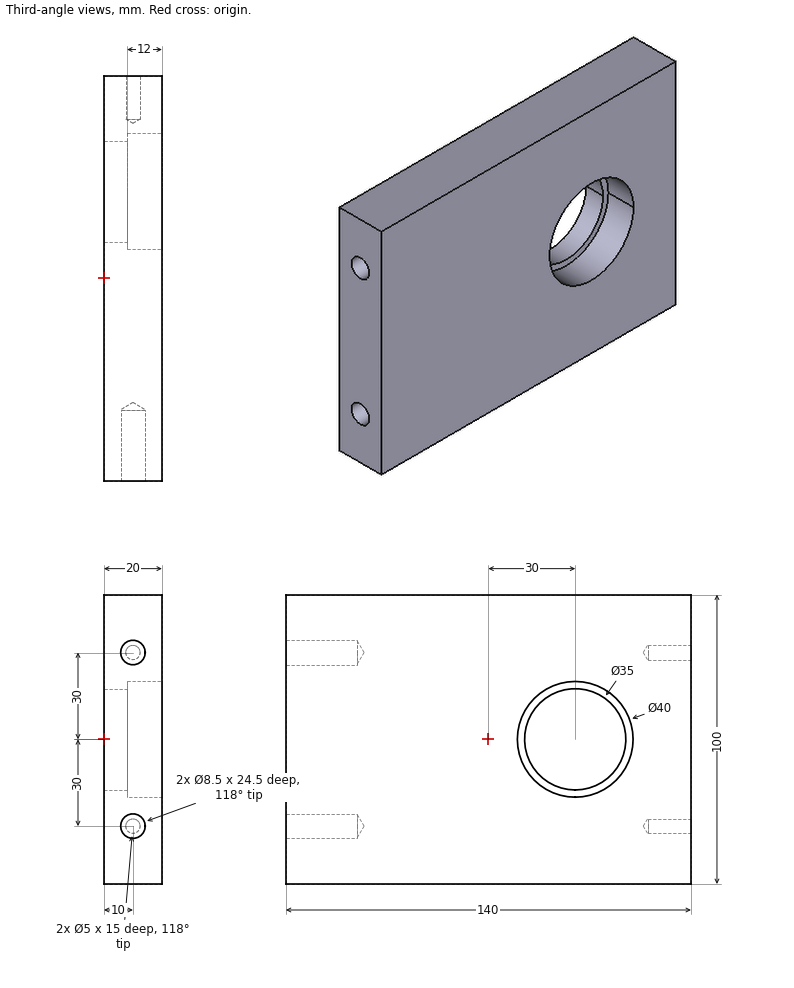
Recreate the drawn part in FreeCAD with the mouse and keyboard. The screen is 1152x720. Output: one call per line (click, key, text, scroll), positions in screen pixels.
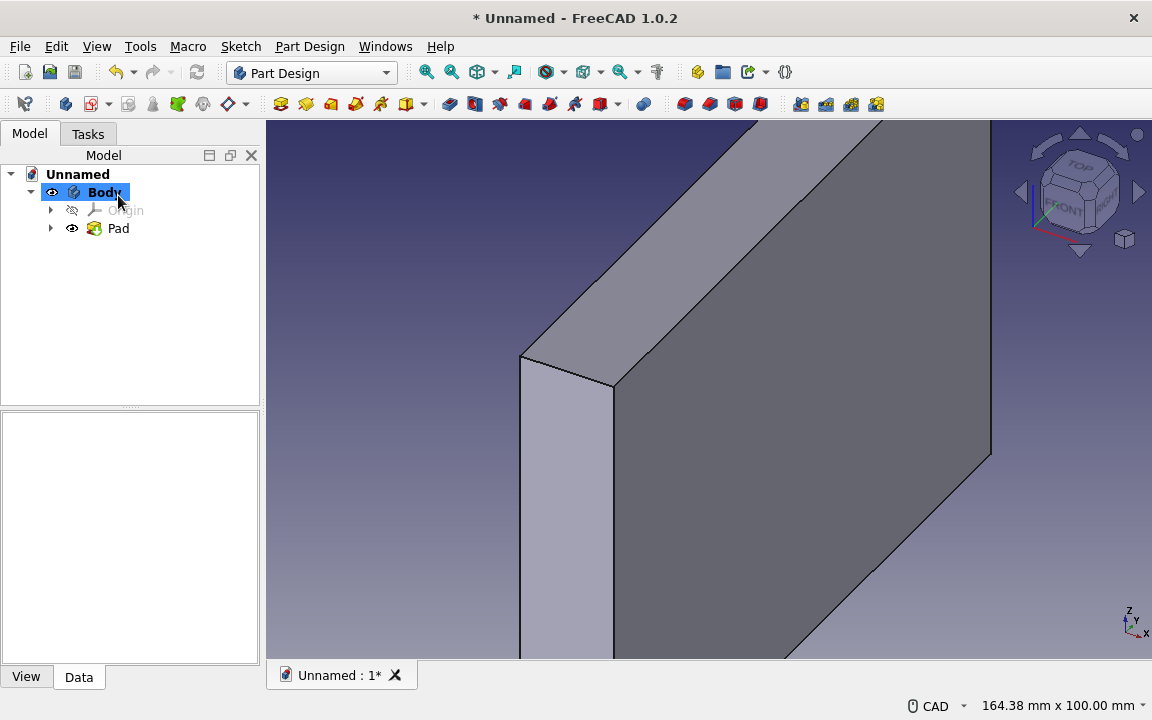
click(427, 72)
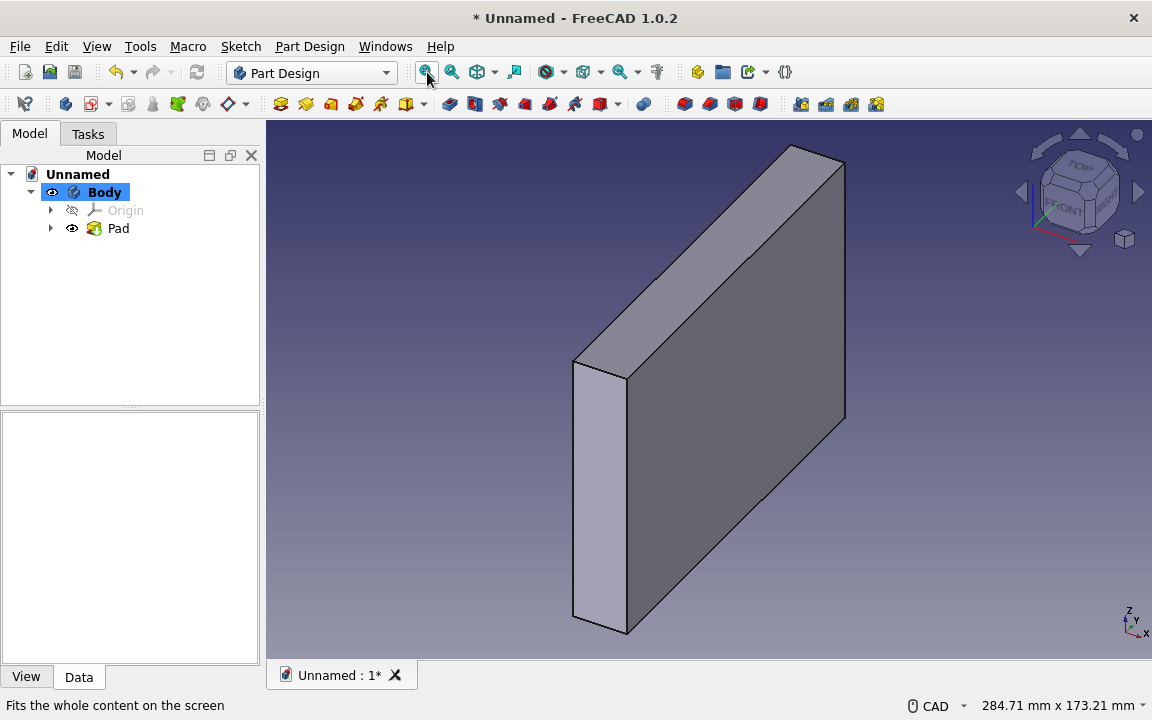
click(600, 497)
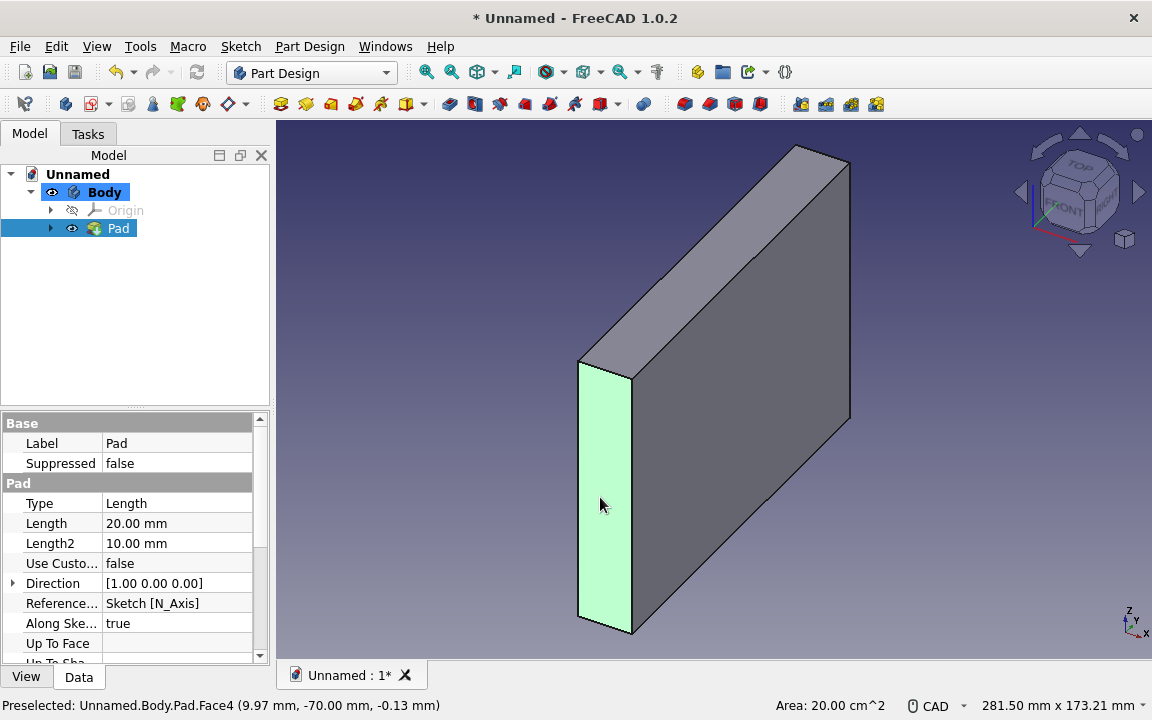
click(90, 104)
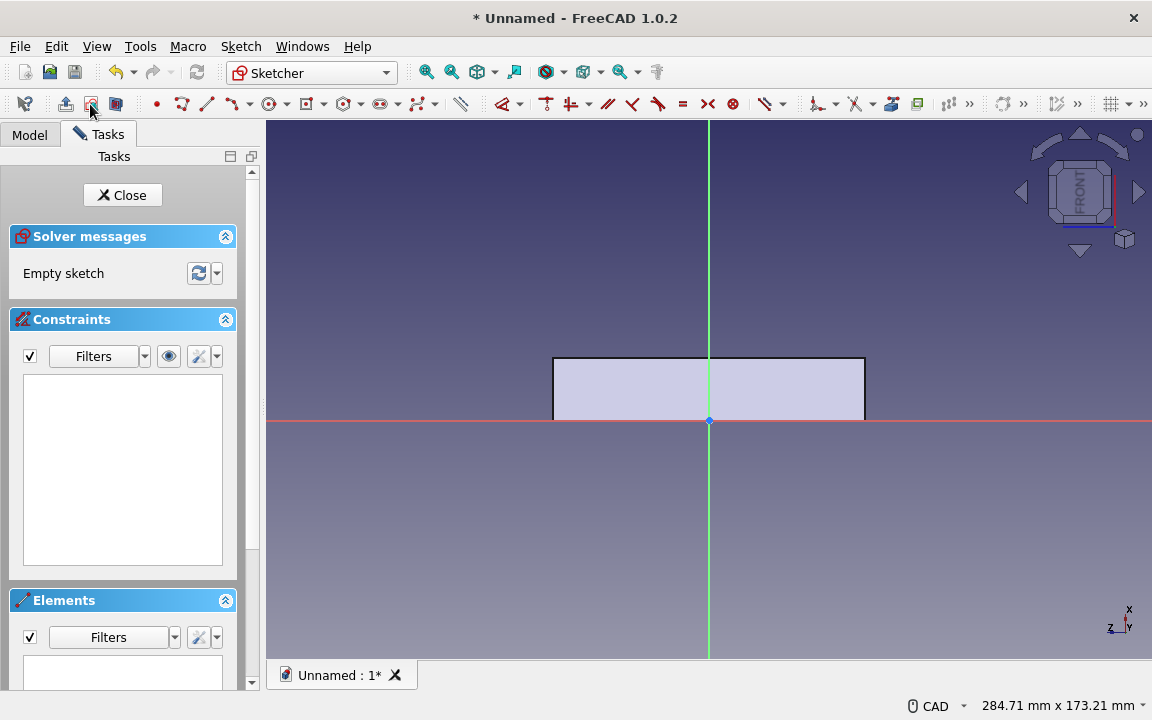
scroll(765, 406, up, 4)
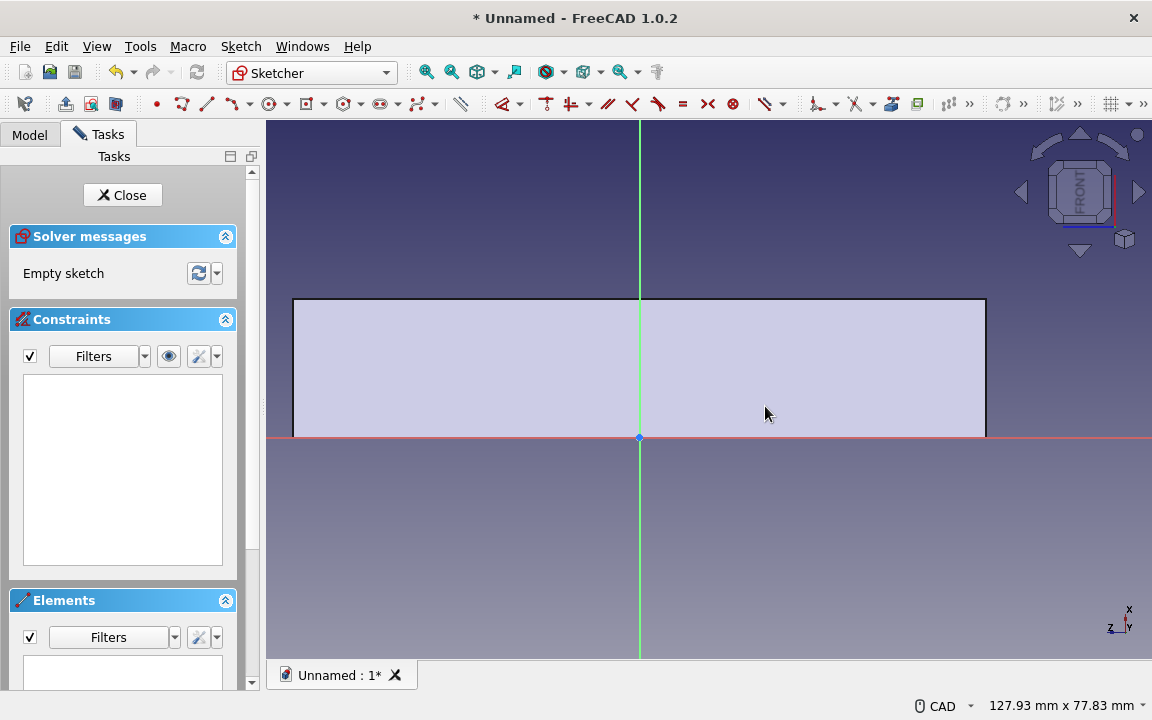
key(g)
key(c)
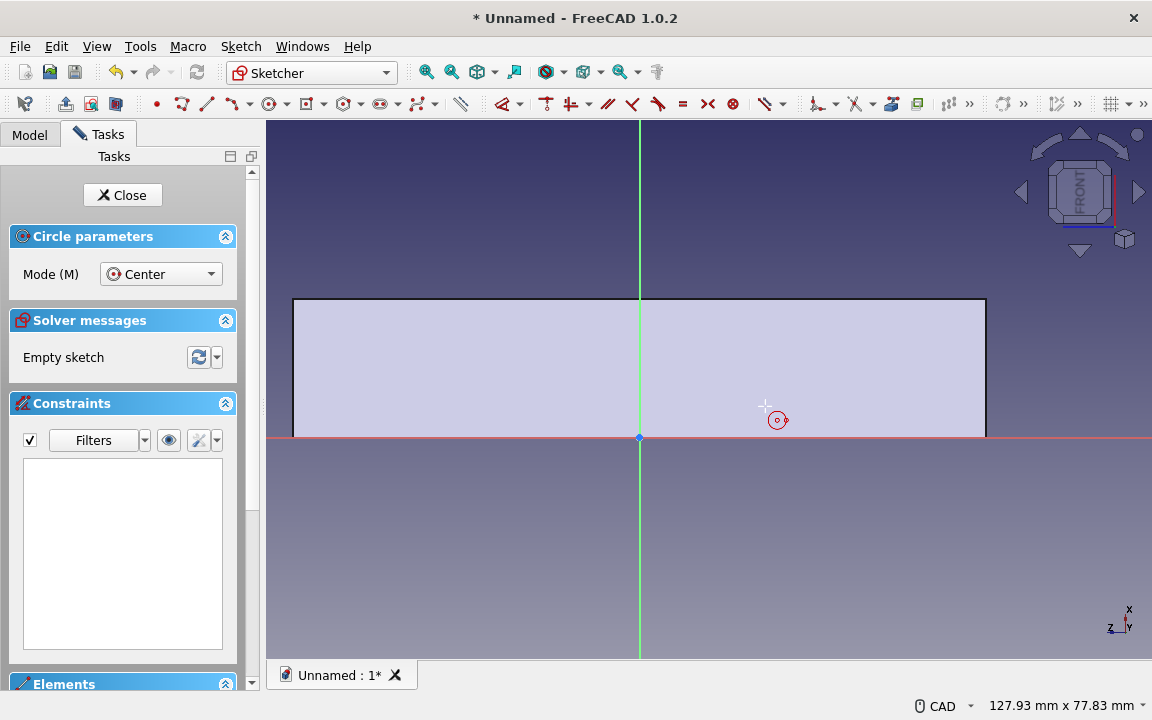
click(847, 369)
move(868, 348)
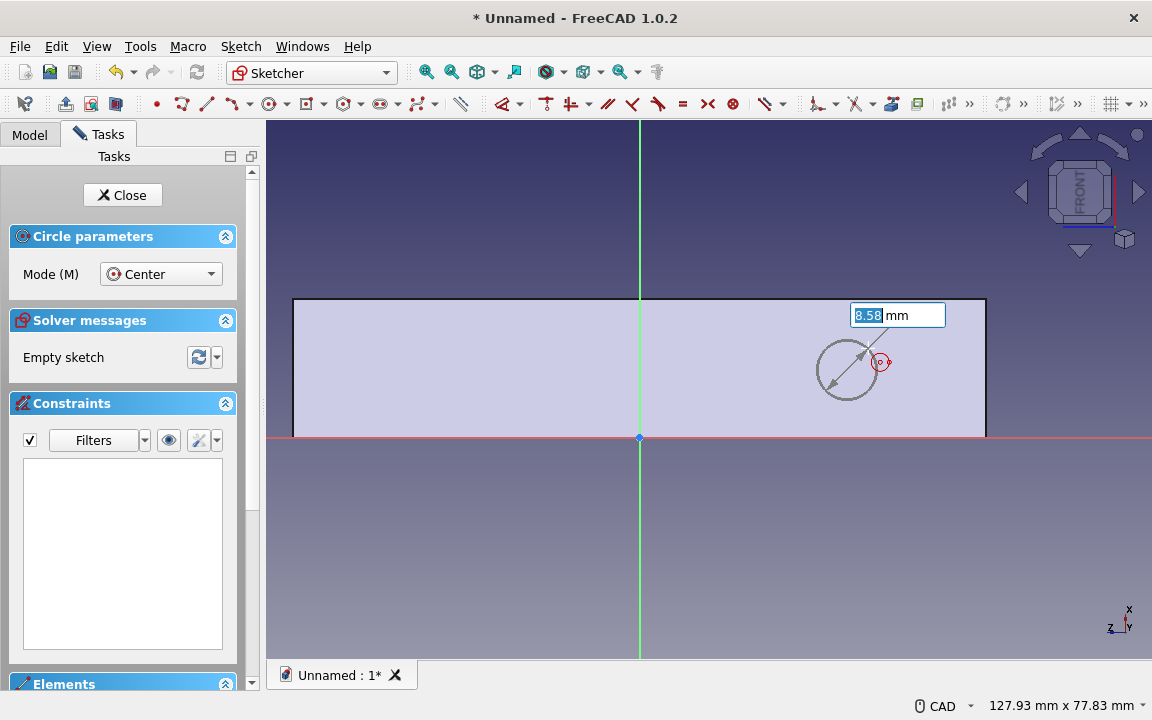
text(8.5)
key(Return)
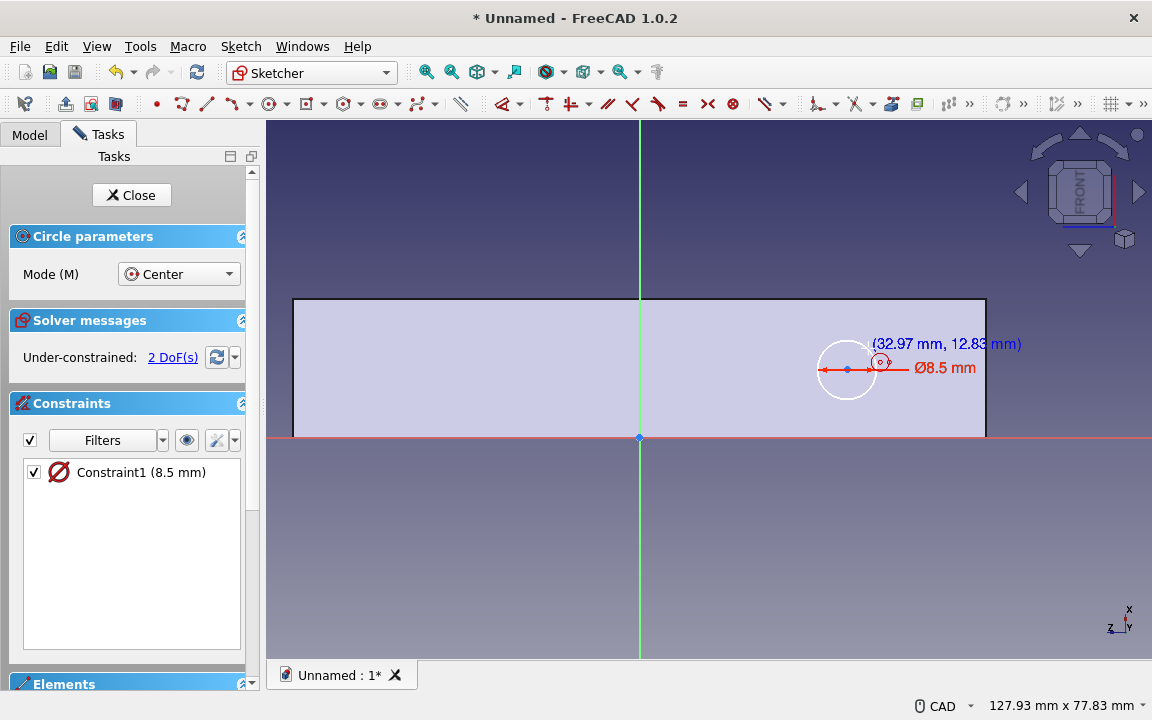
click(432, 369)
move(453, 348)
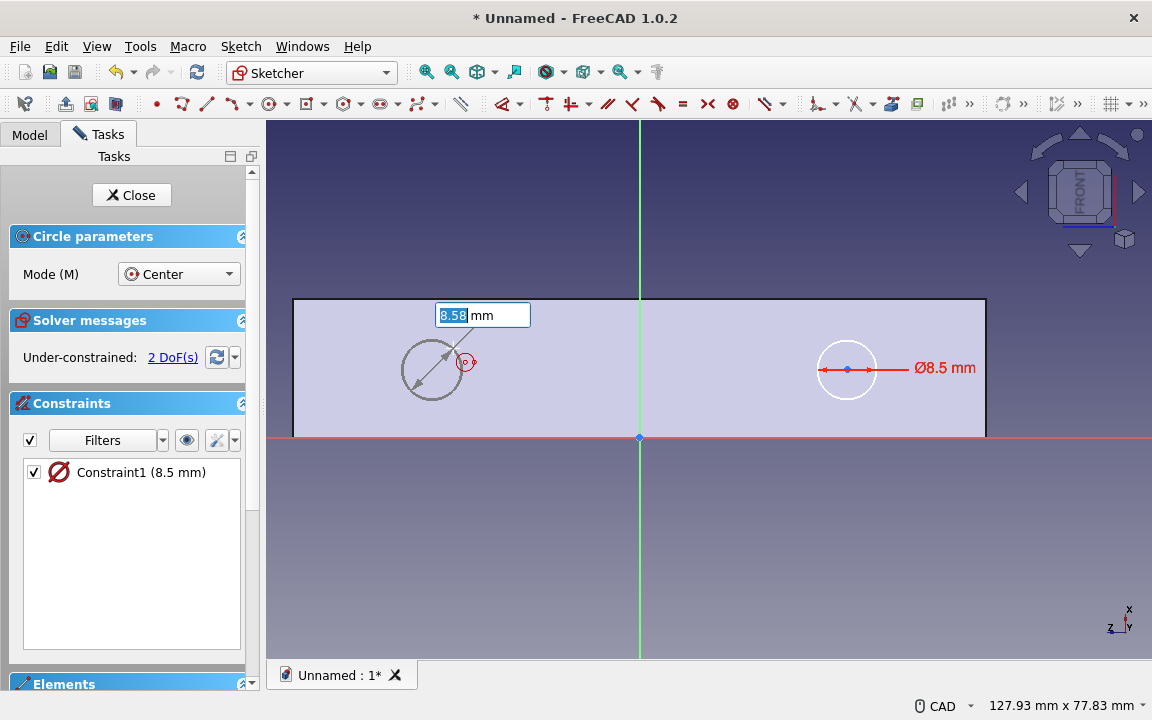
text(8.5)
key(Return)
key(Escape)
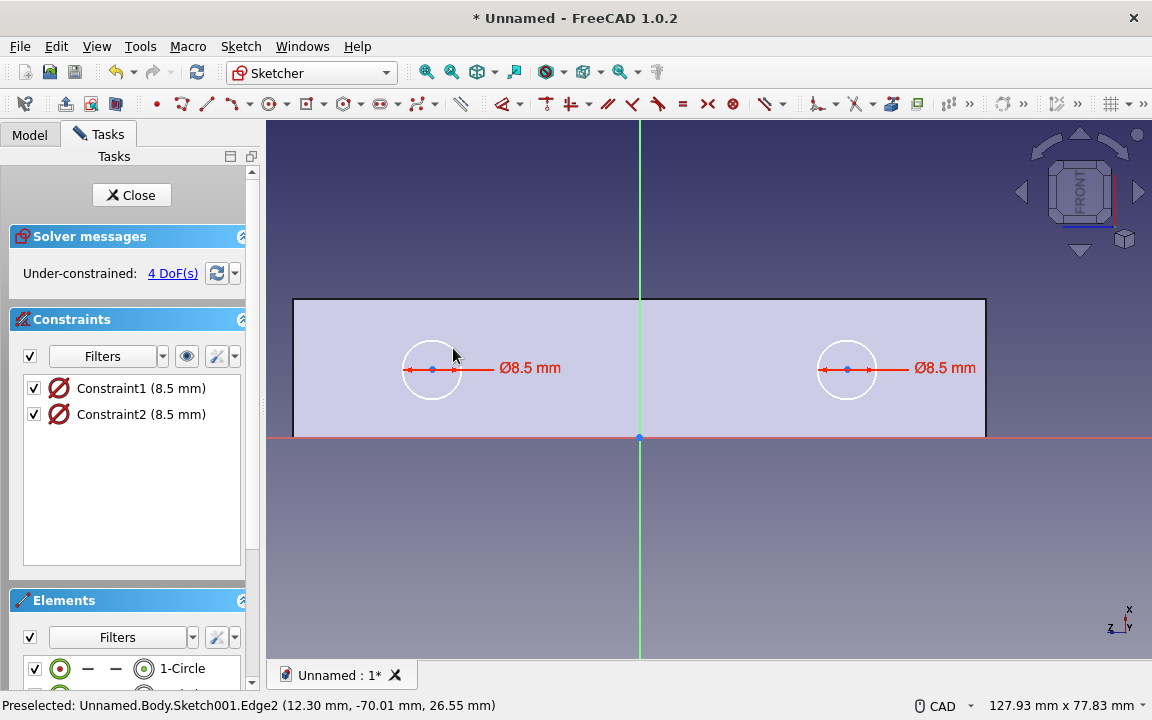
click(847, 370)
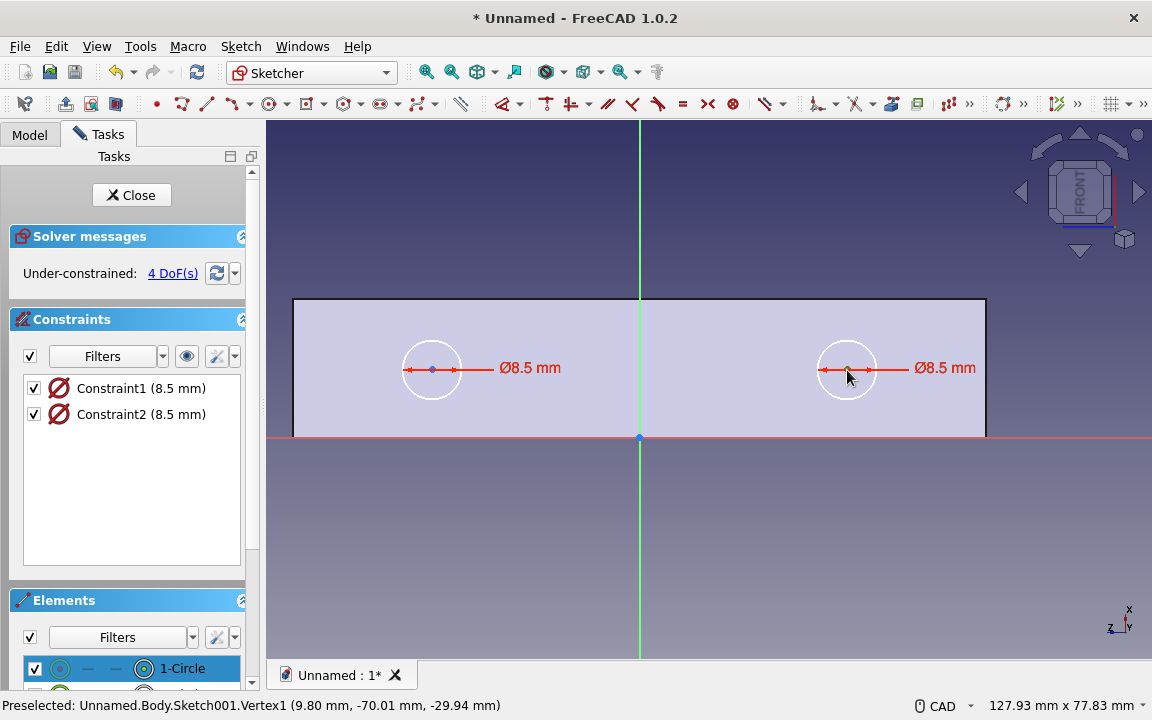
click(432, 370)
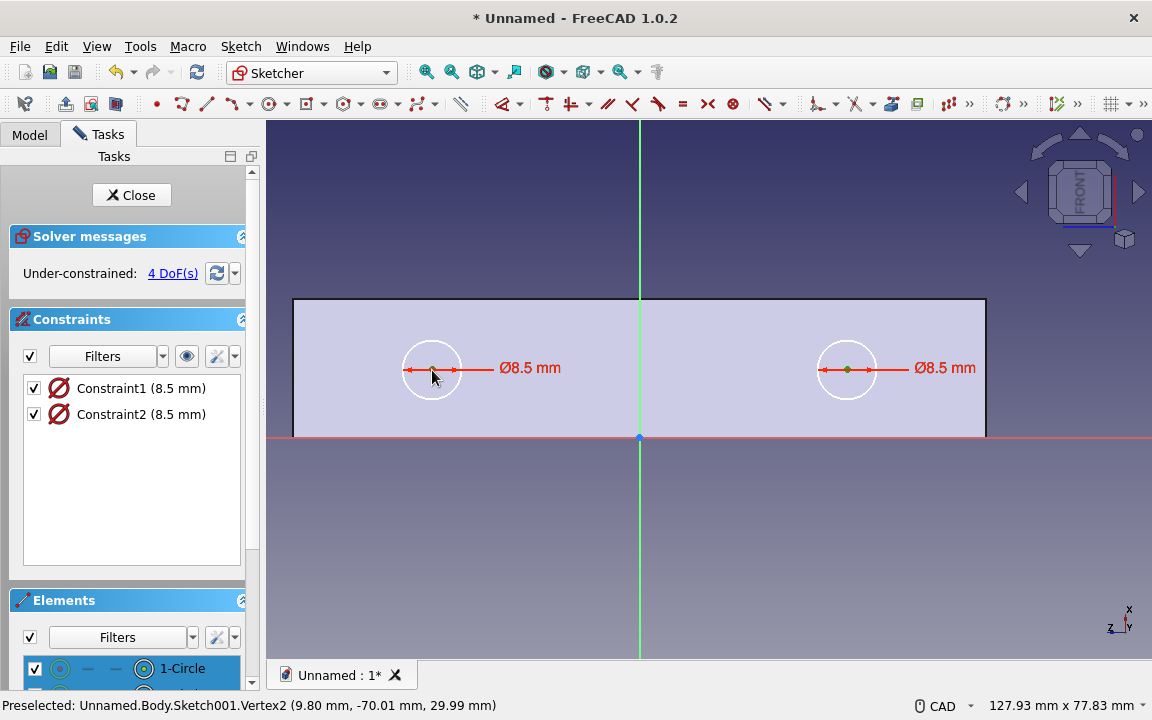
key(h)